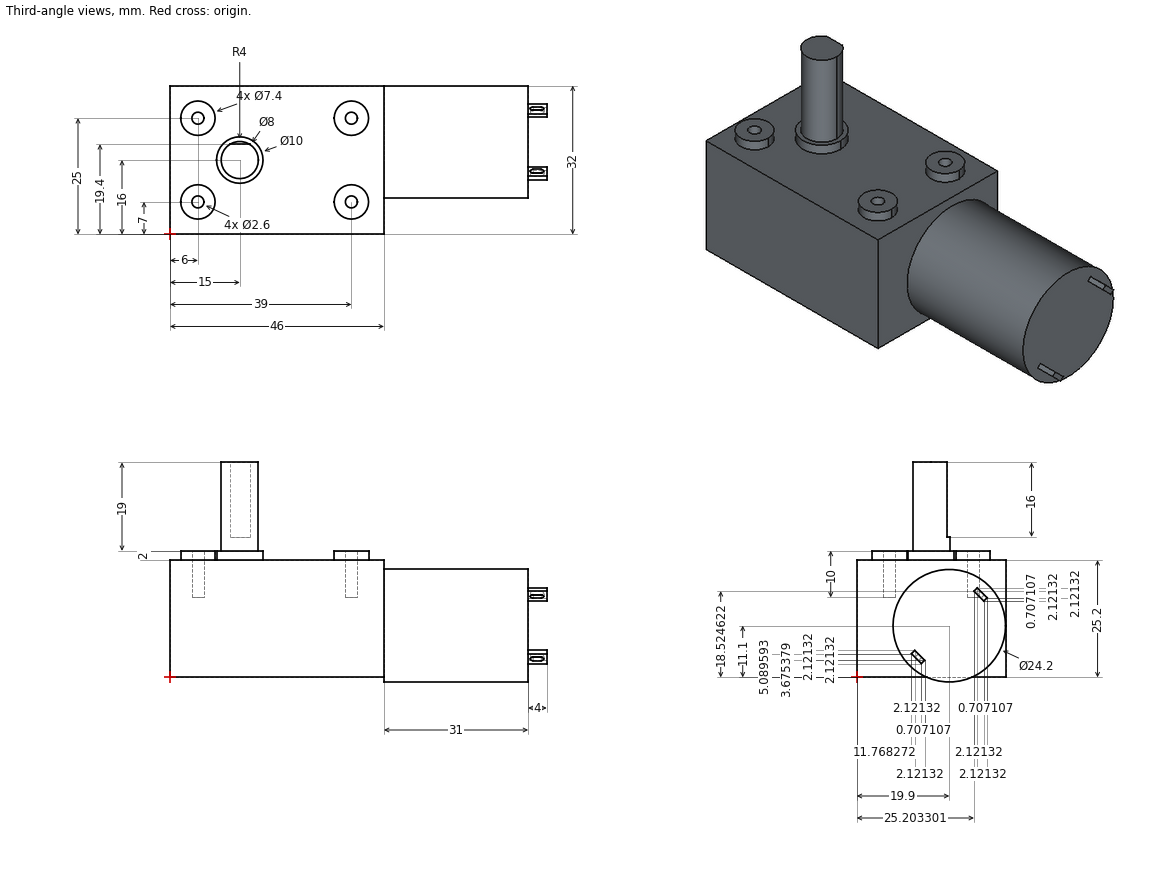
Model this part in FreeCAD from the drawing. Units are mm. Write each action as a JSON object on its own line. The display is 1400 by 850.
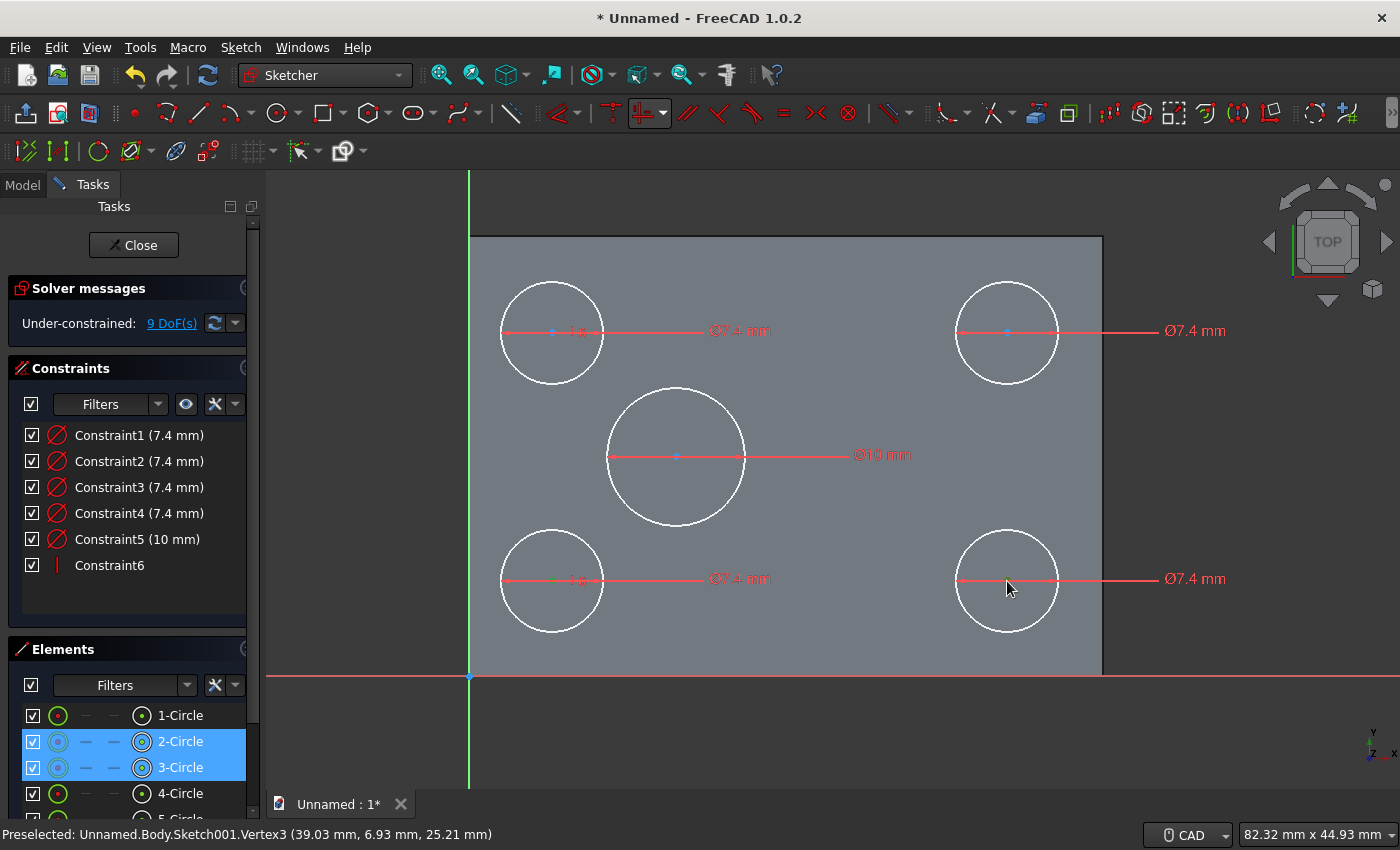
{"action": "key", "text": "h"}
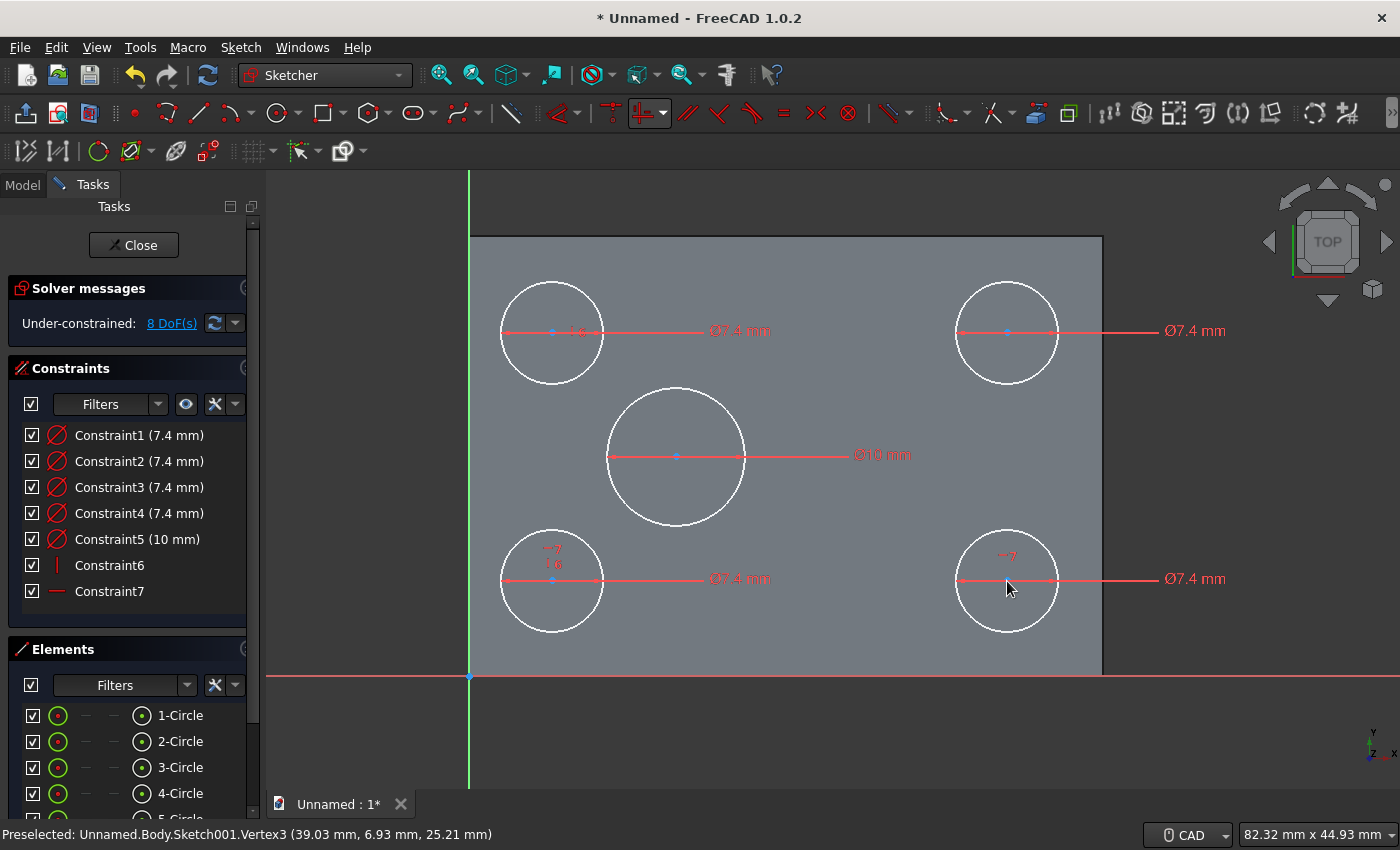
{"action": "left_click", "coordinate": [1007, 581]}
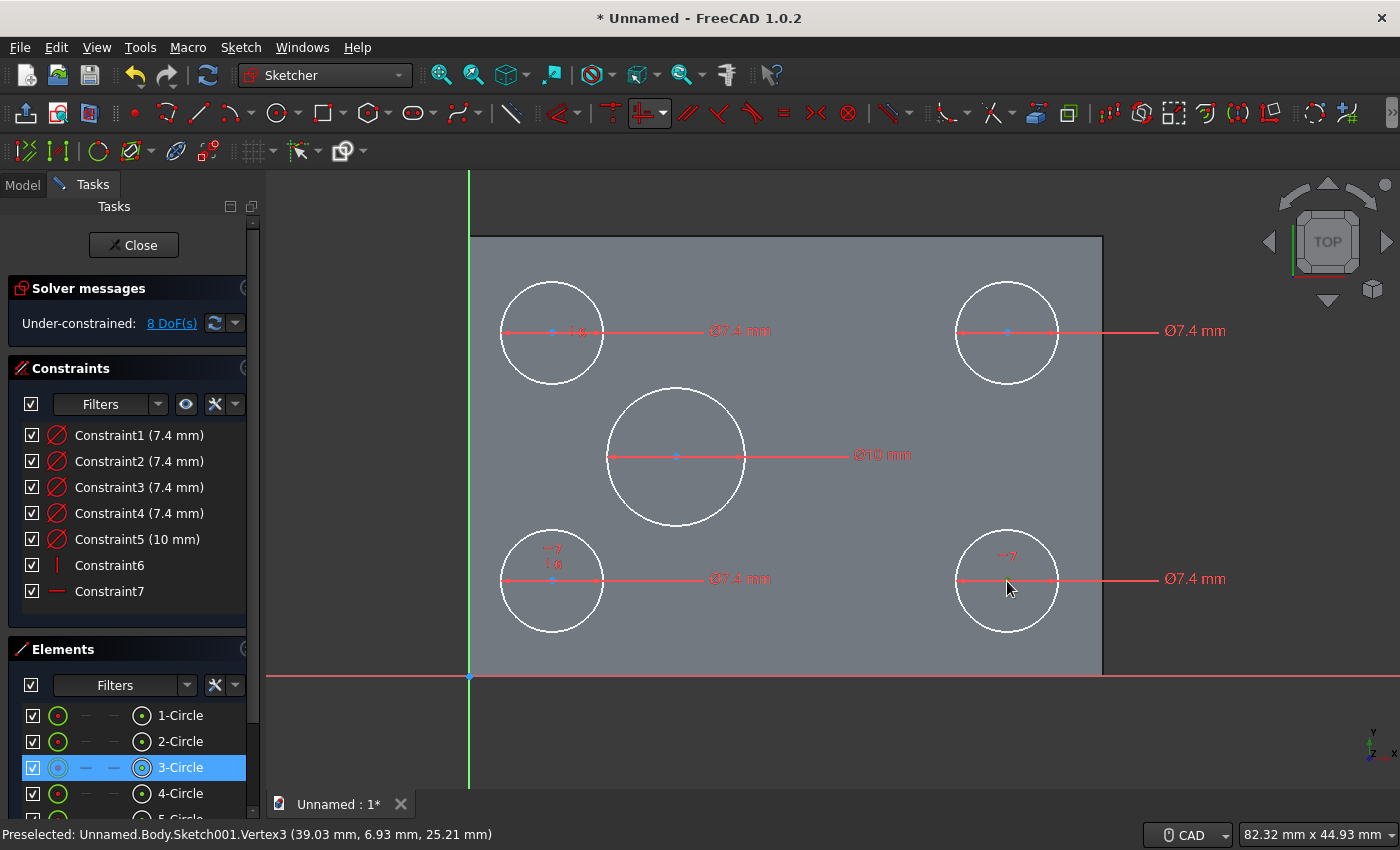
{"action": "left_click", "coordinate": [1007, 333]}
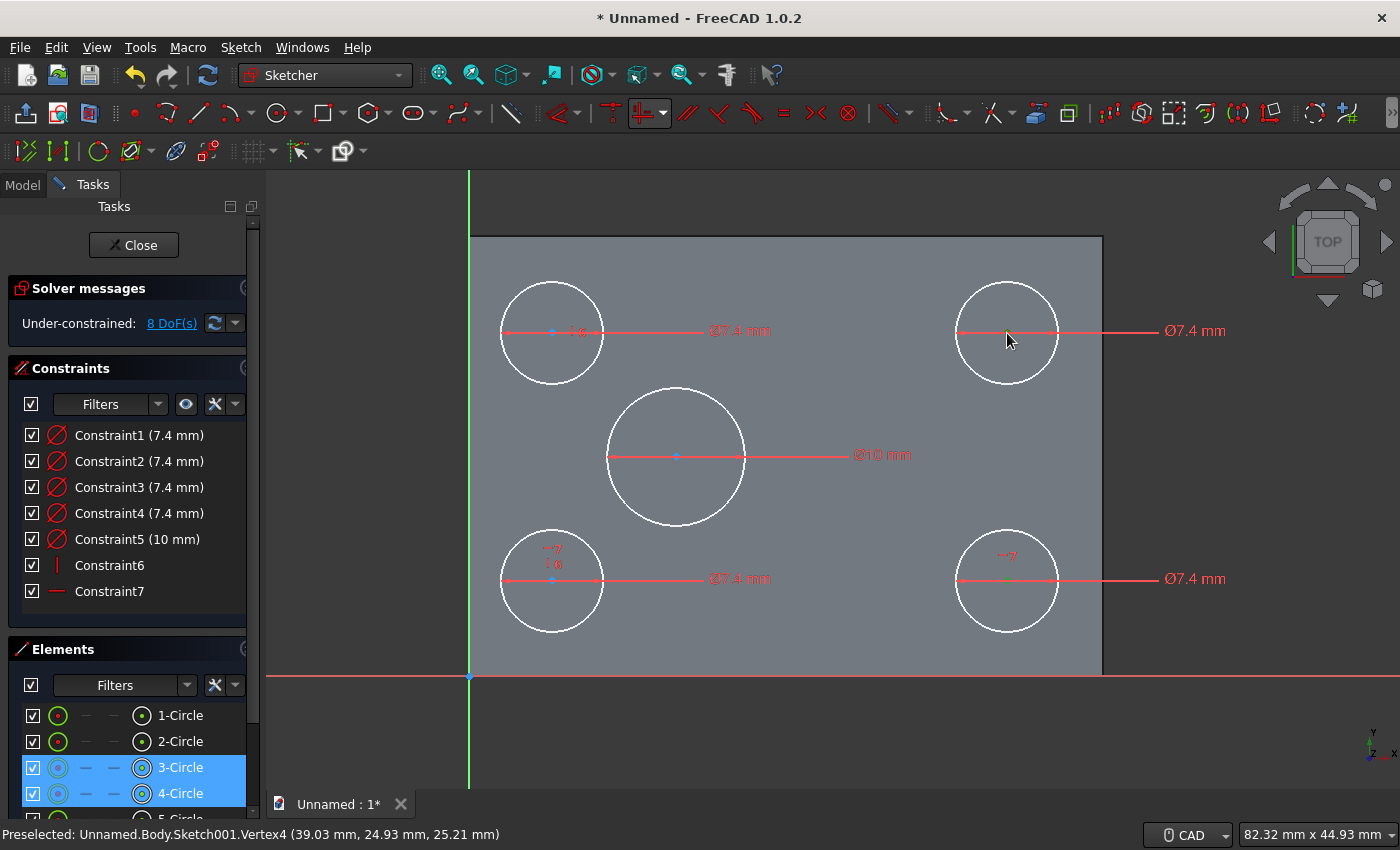
{"action": "left_click", "coordinate": [666, 114]}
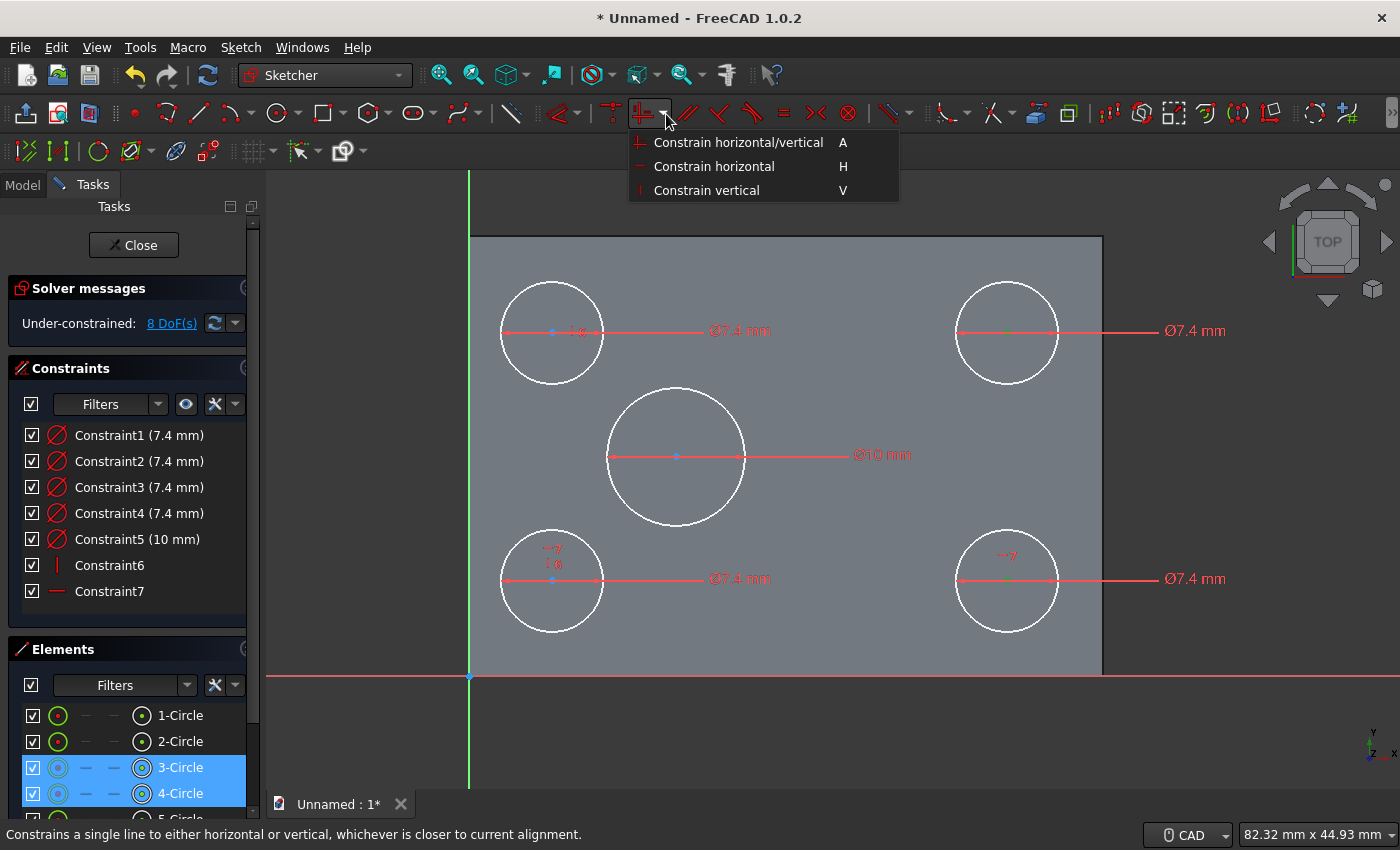
{"action": "left_click", "coordinate": [764, 190]}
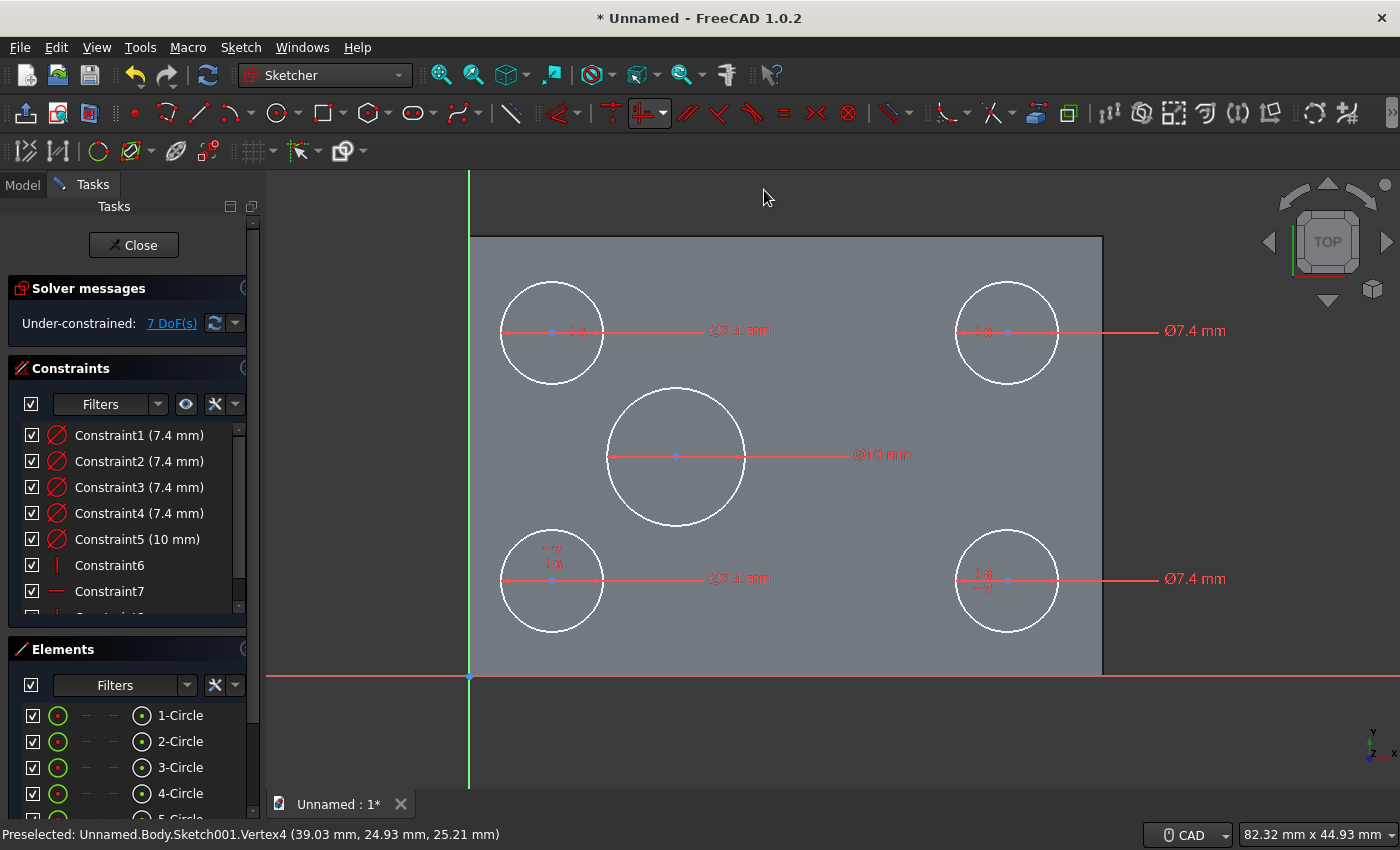
{"action": "left_click", "coordinate": [552, 333]}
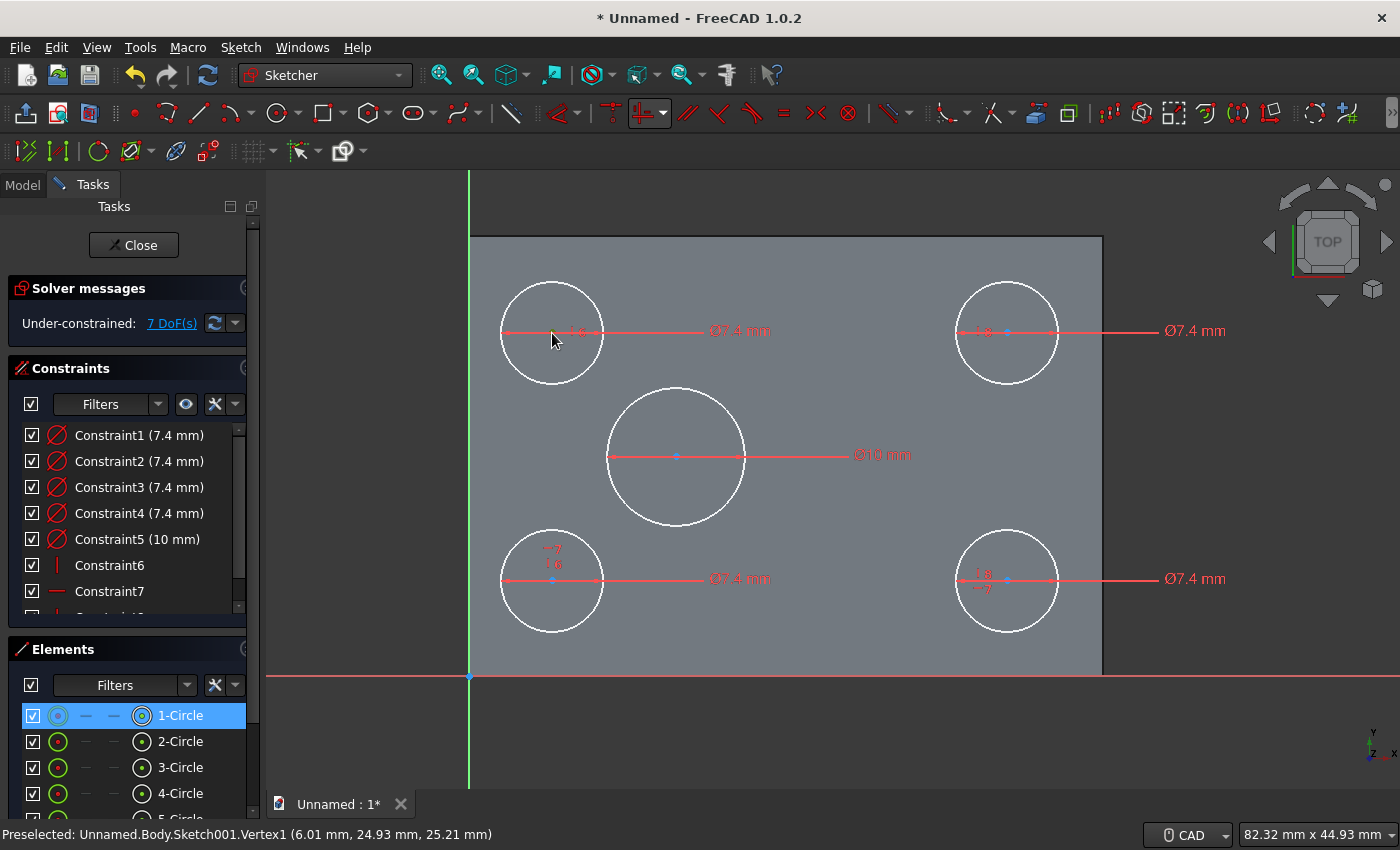
{"action": "left_click", "coordinate": [1007, 333]}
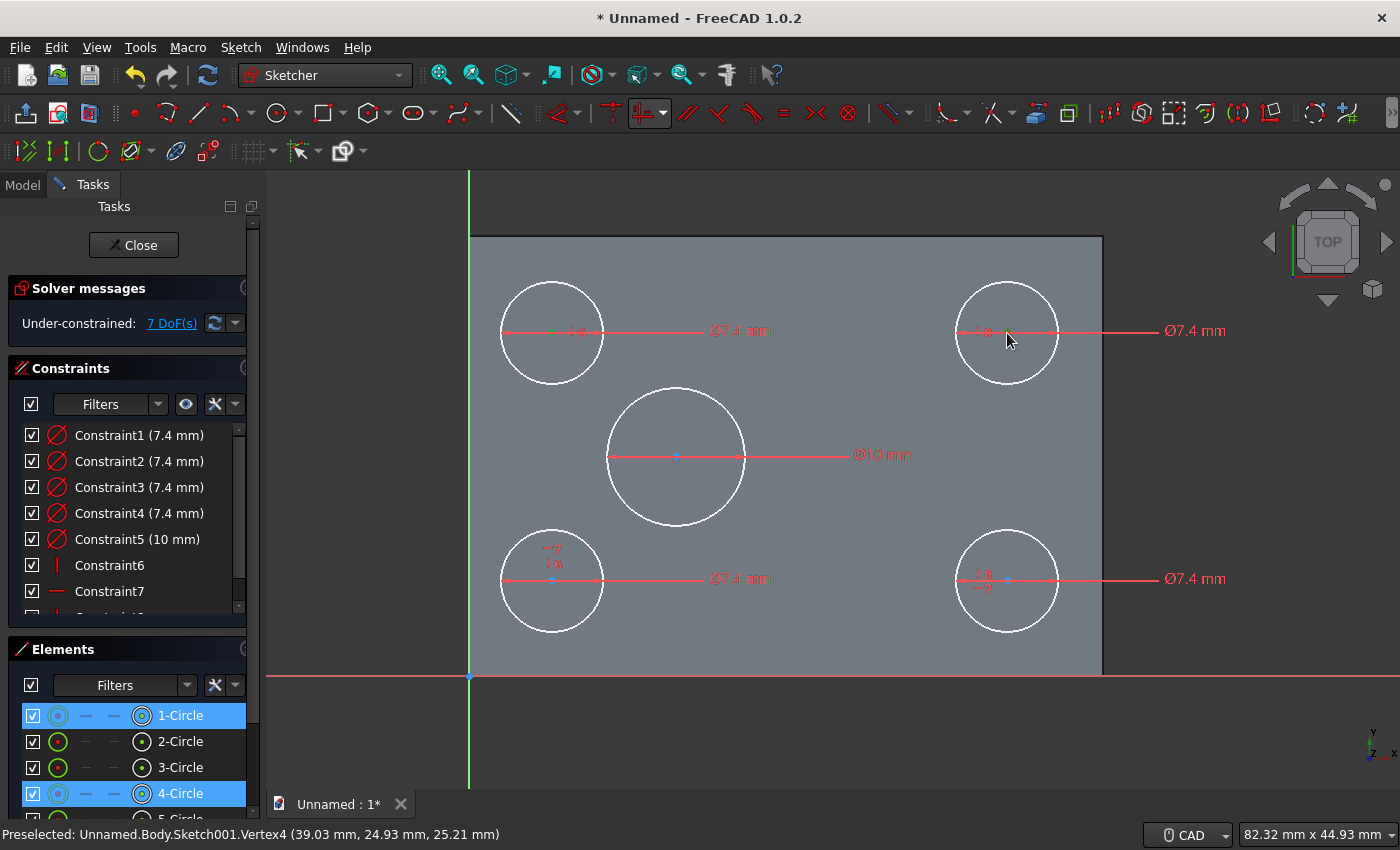
{"action": "left_click", "coordinate": [666, 114]}